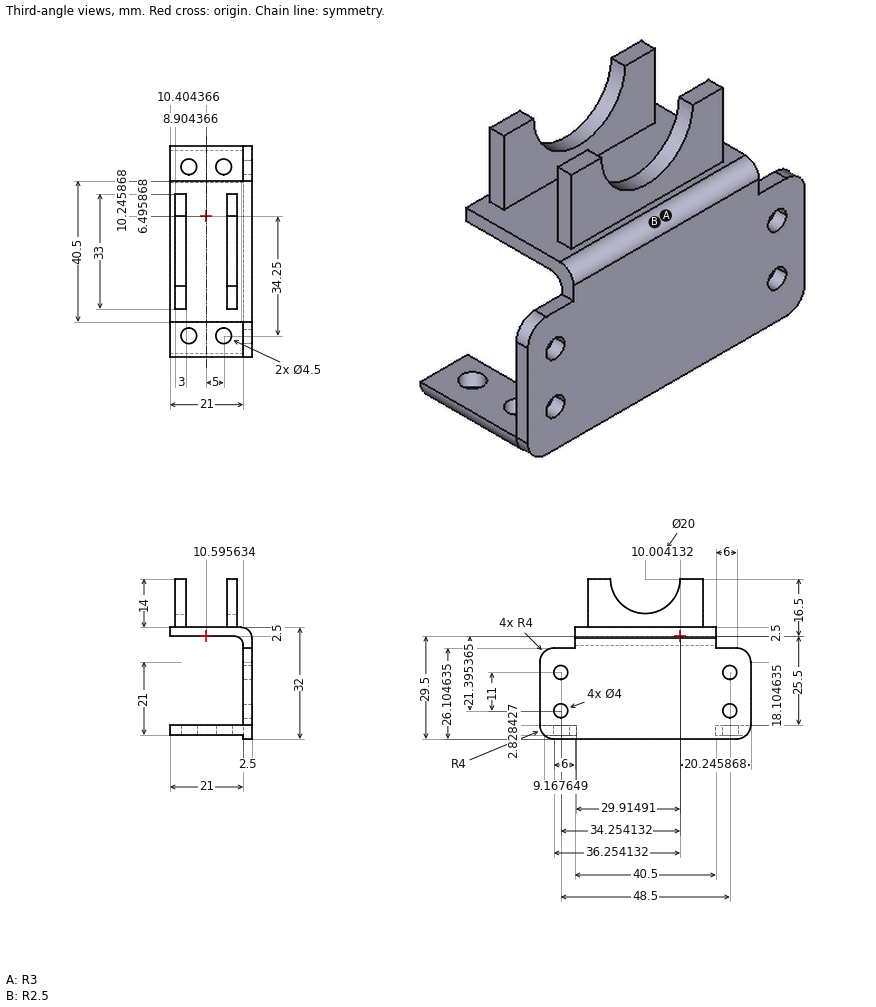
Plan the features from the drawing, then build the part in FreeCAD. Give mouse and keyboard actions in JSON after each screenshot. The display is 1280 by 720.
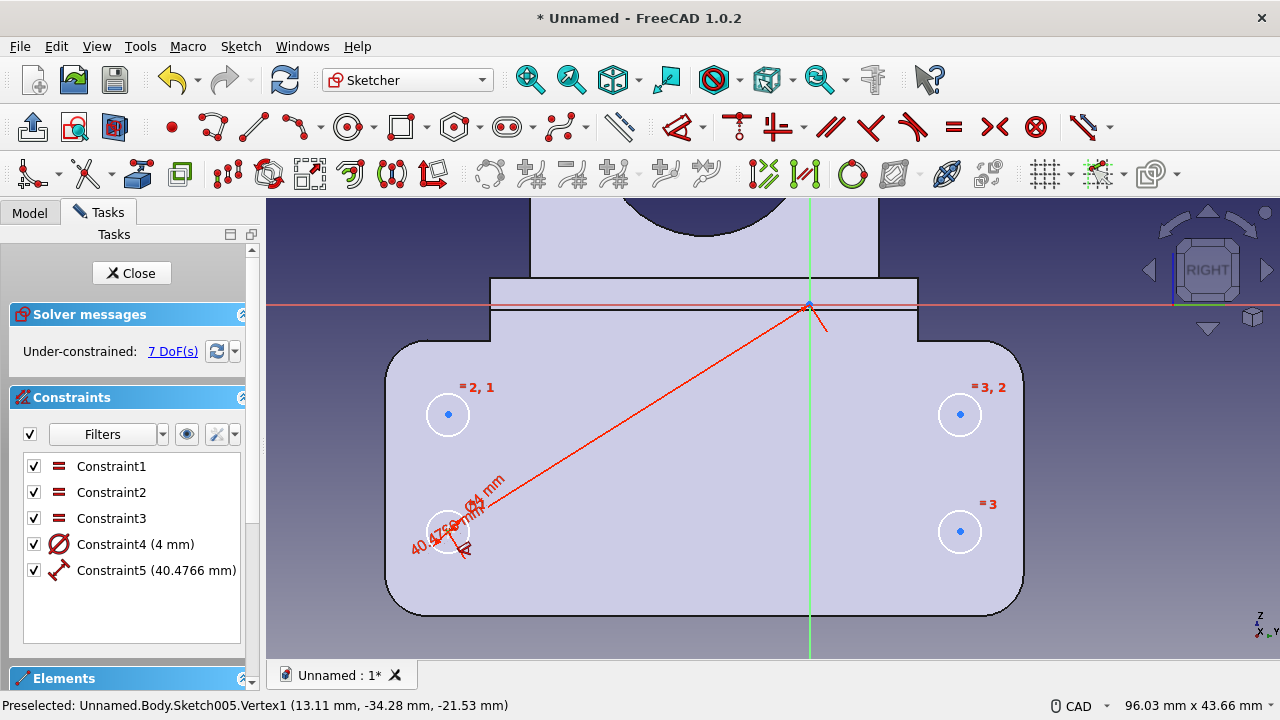
{"action": "left_click", "coordinate": [448, 415]}
{"action": "left_click", "coordinate": [414, 473]}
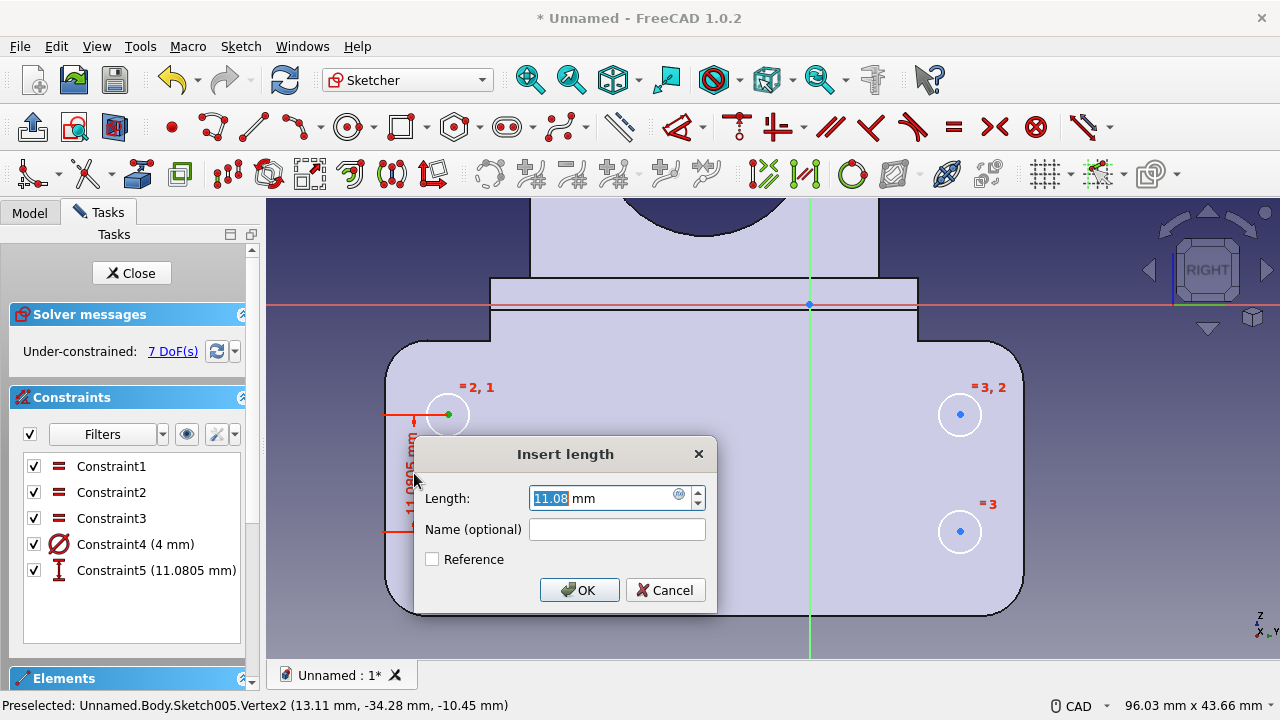
{"action": "type", "text": "11"}
{"action": "key", "text": "Return"}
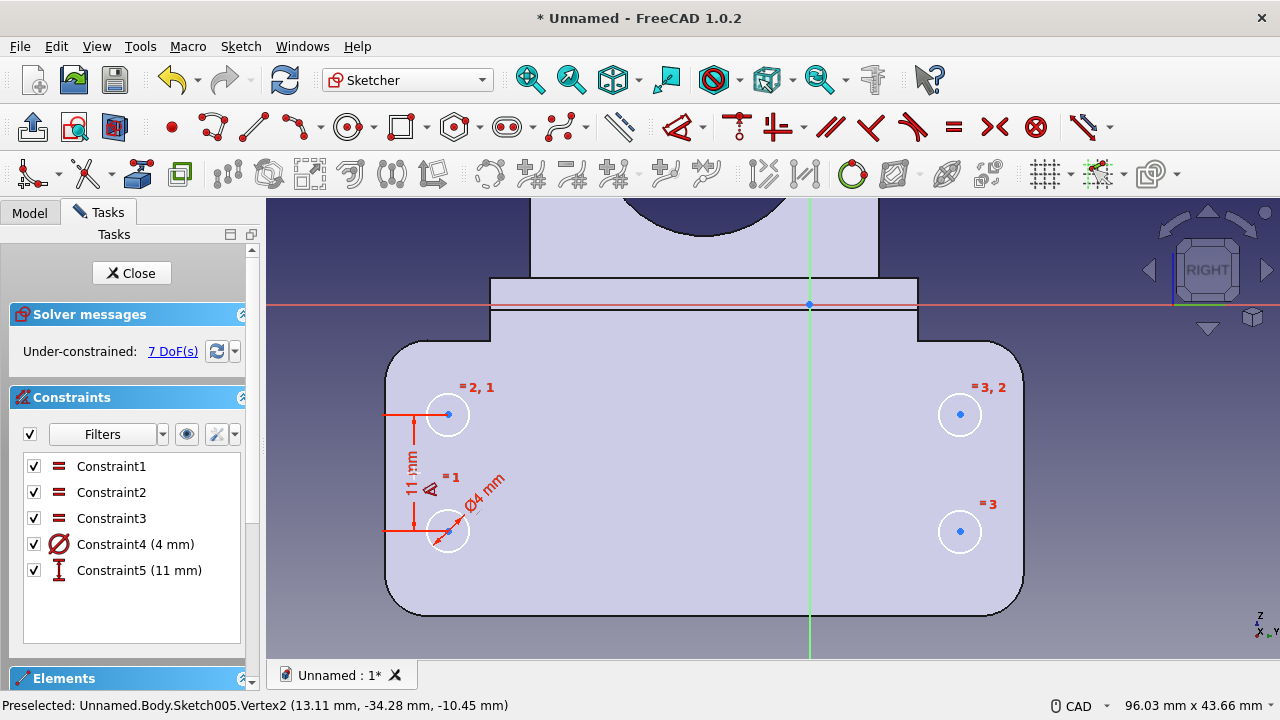
{"action": "left_click", "coordinate": [448, 531]}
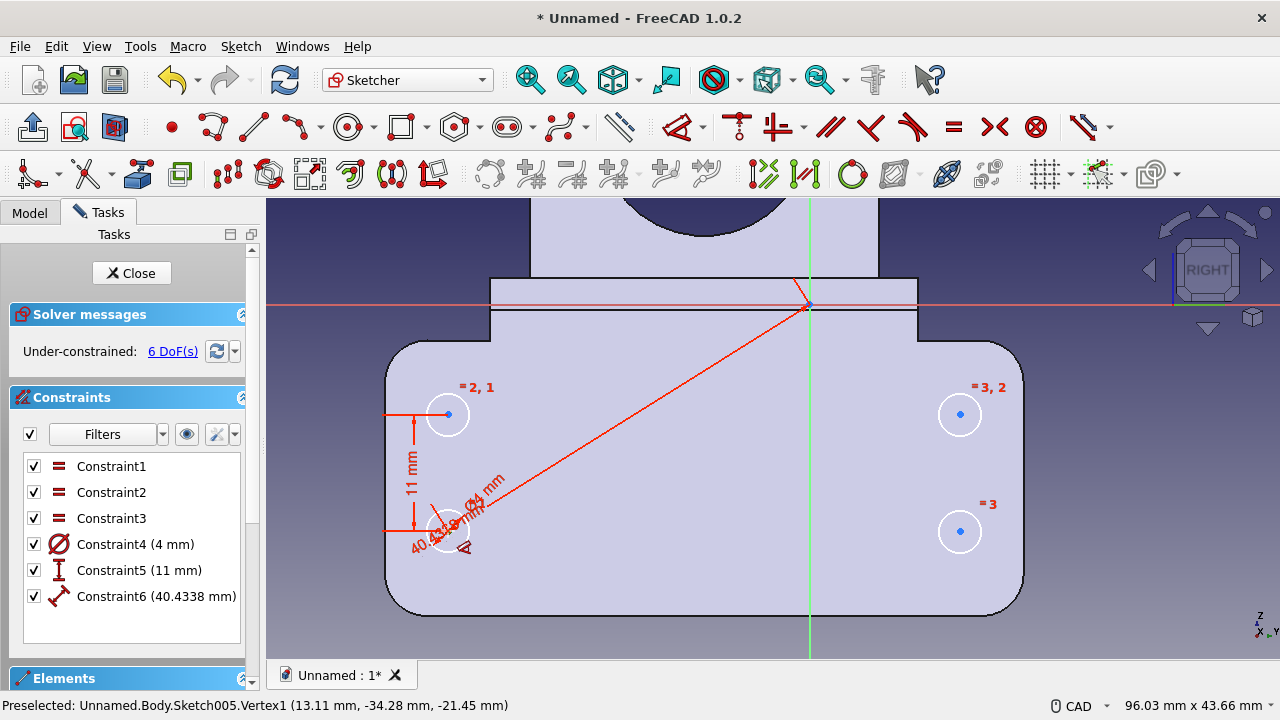
{"action": "left_click", "coordinate": [960, 415]}
{"action": "left_click", "coordinate": [414, 446]}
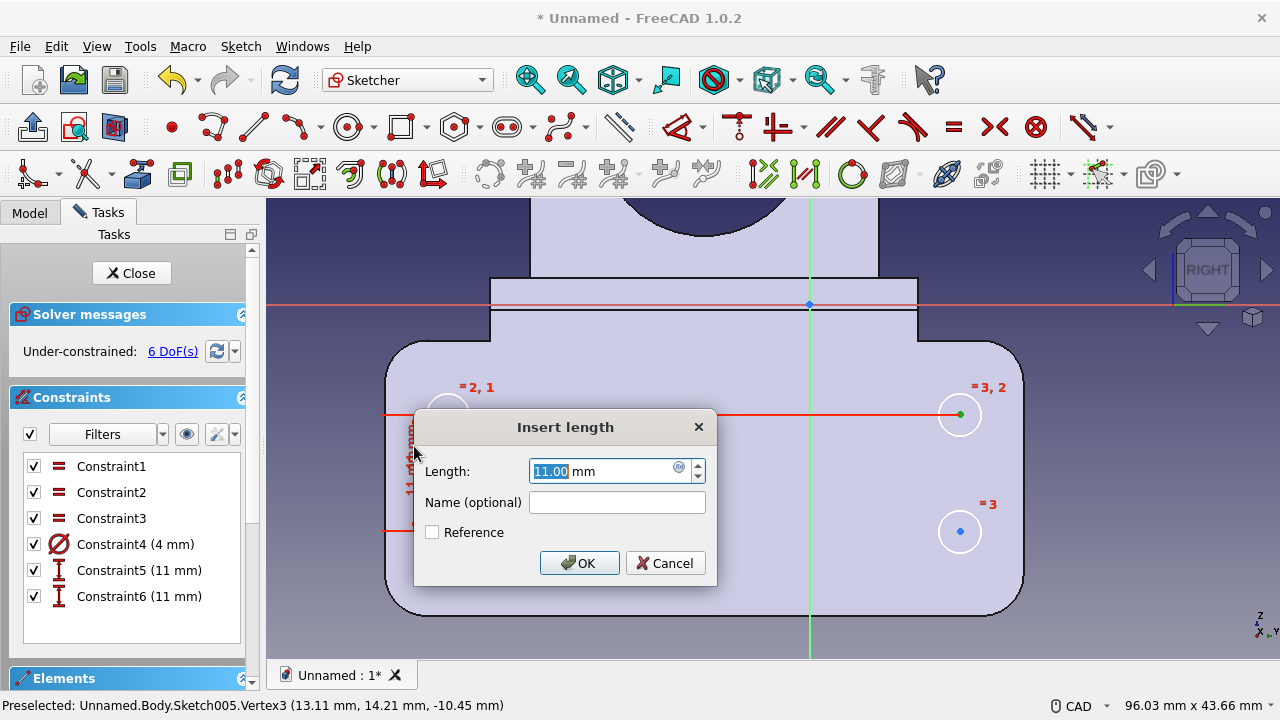
{"action": "type", "text": "11"}
{"action": "key", "text": "Return"}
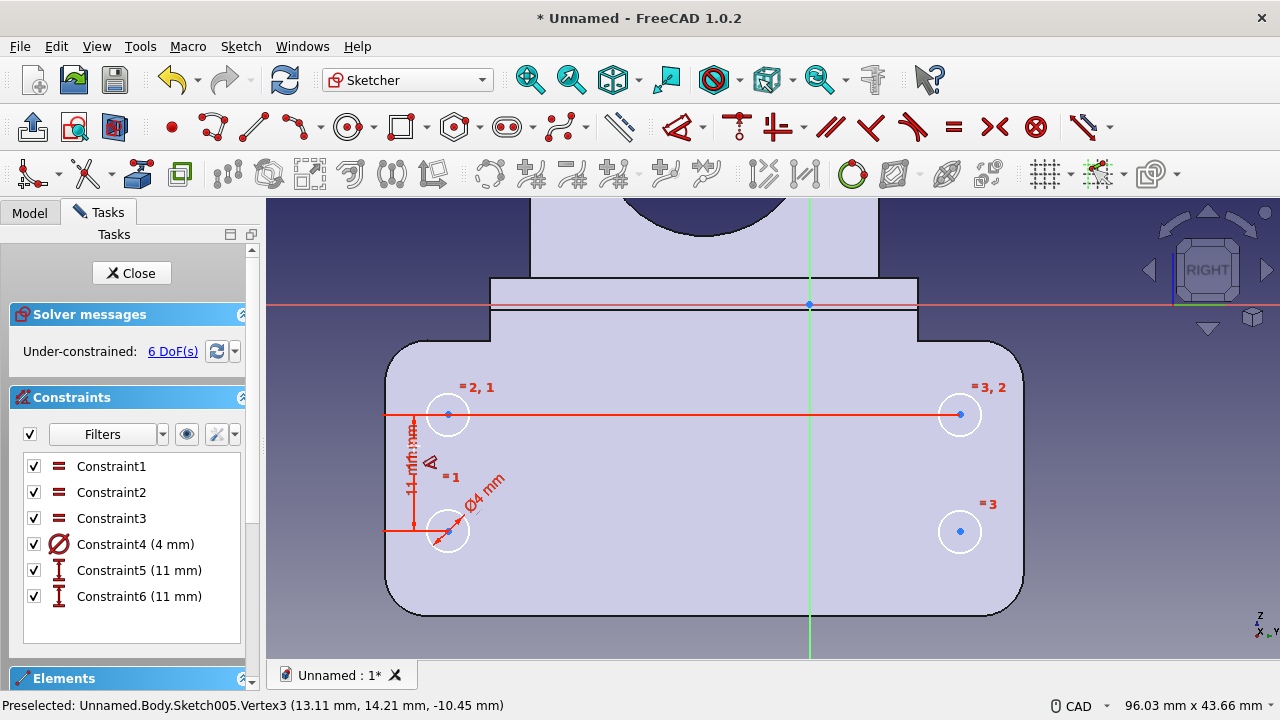
{"action": "left_click", "coordinate": [960, 415]}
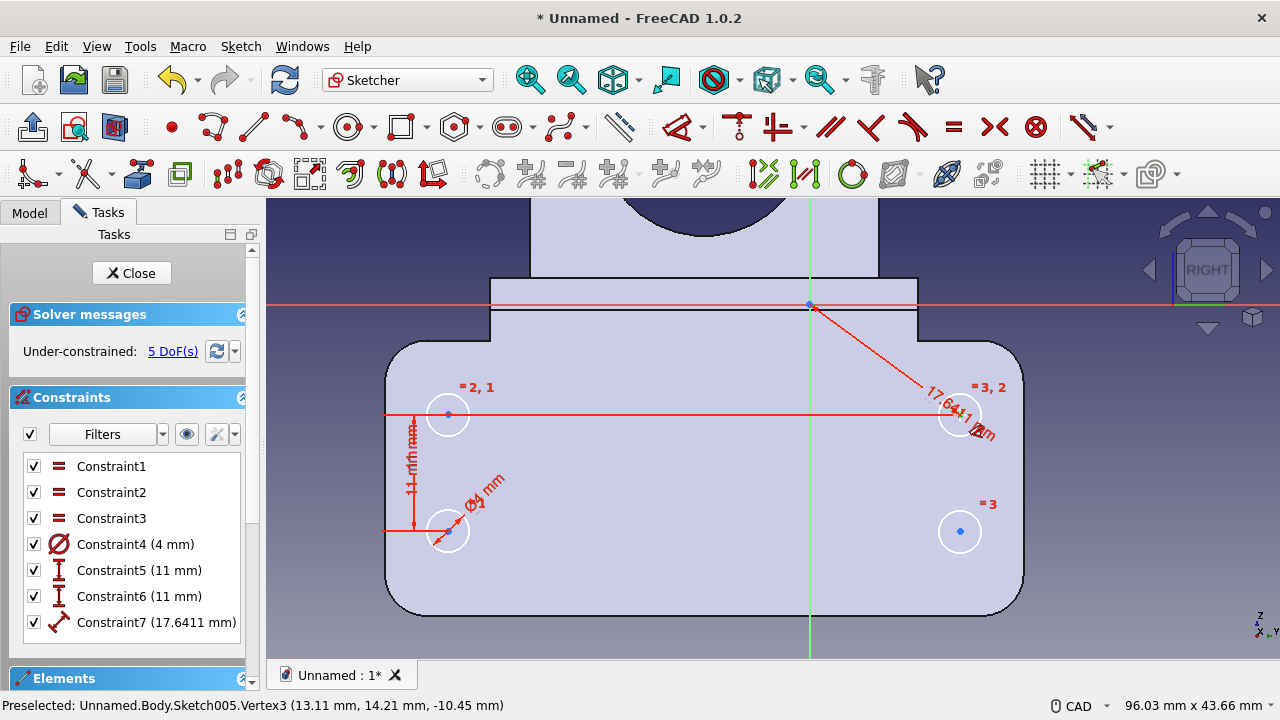
{"action": "left_click", "coordinate": [960, 532]}
{"action": "left_click", "coordinate": [994, 473]}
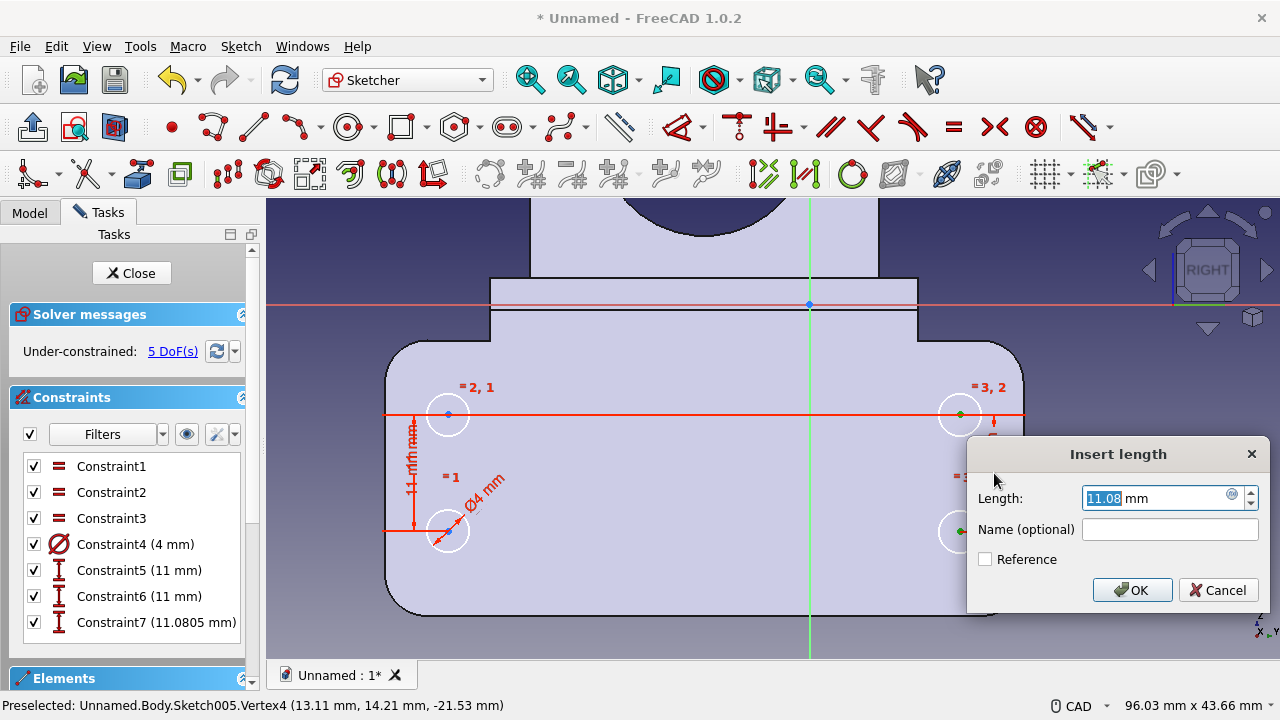
{"action": "type", "text": "11"}
{"action": "key", "text": "Return"}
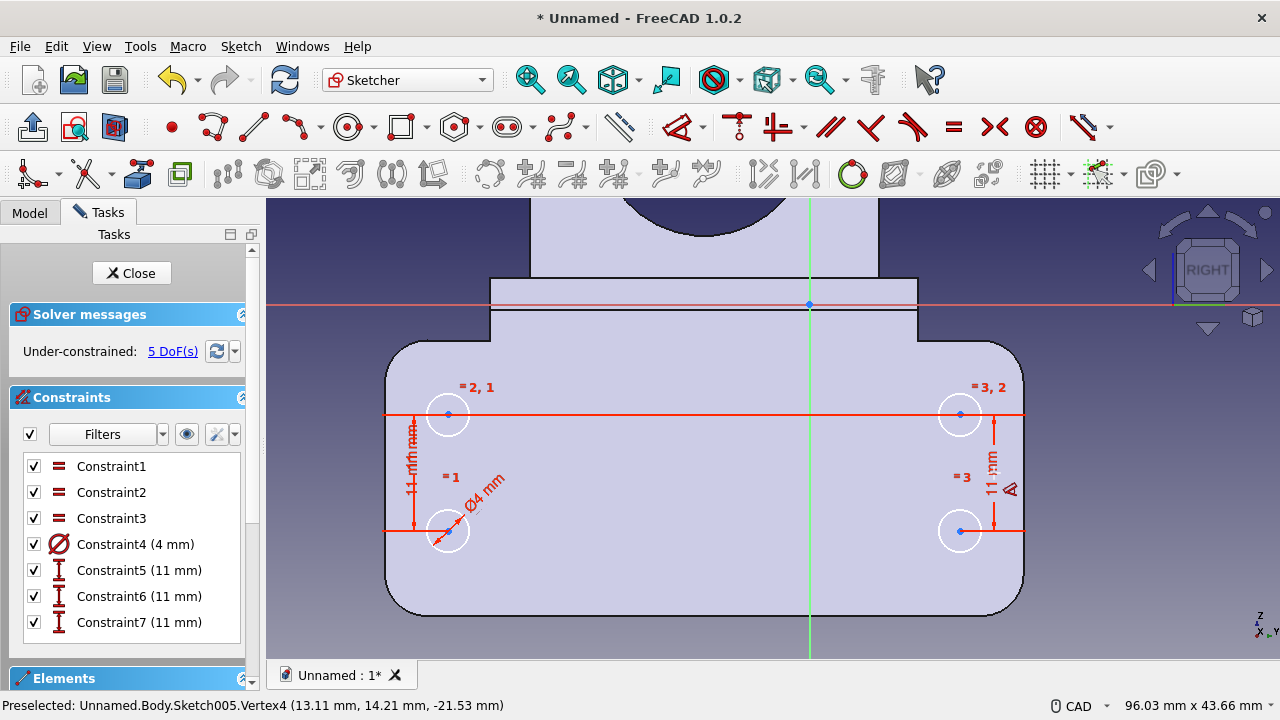
{"action": "left_click", "coordinate": [448, 415]}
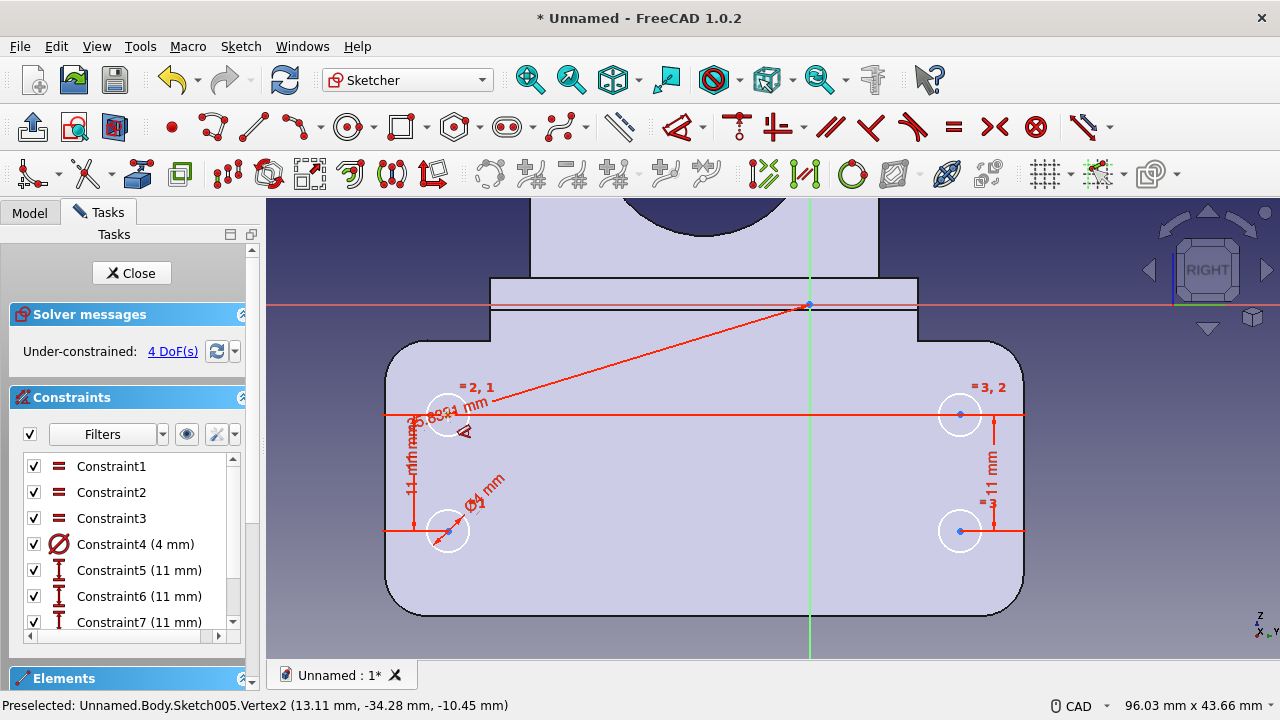
{"action": "left_click", "coordinate": [960, 415]}
{"action": "left_click", "coordinate": [704, 381]}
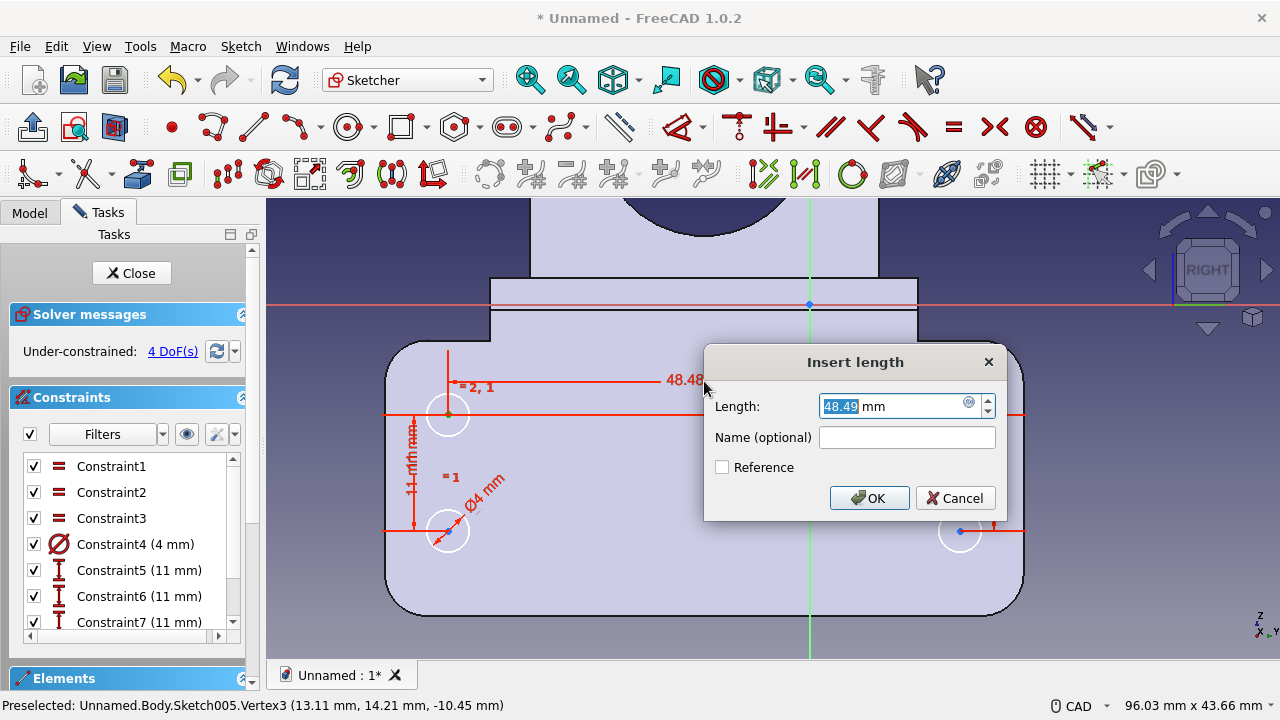
{"action": "type", "text": "48.5"}
{"action": "key", "text": "Return"}